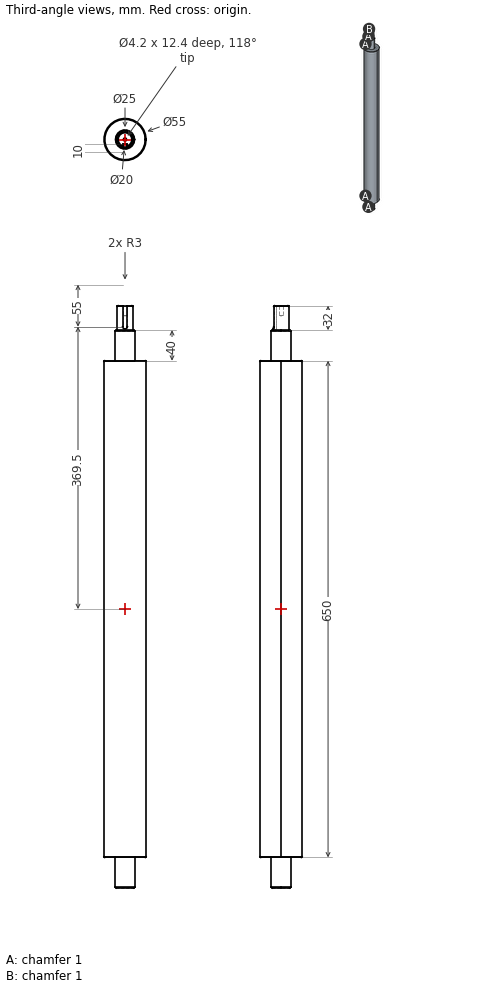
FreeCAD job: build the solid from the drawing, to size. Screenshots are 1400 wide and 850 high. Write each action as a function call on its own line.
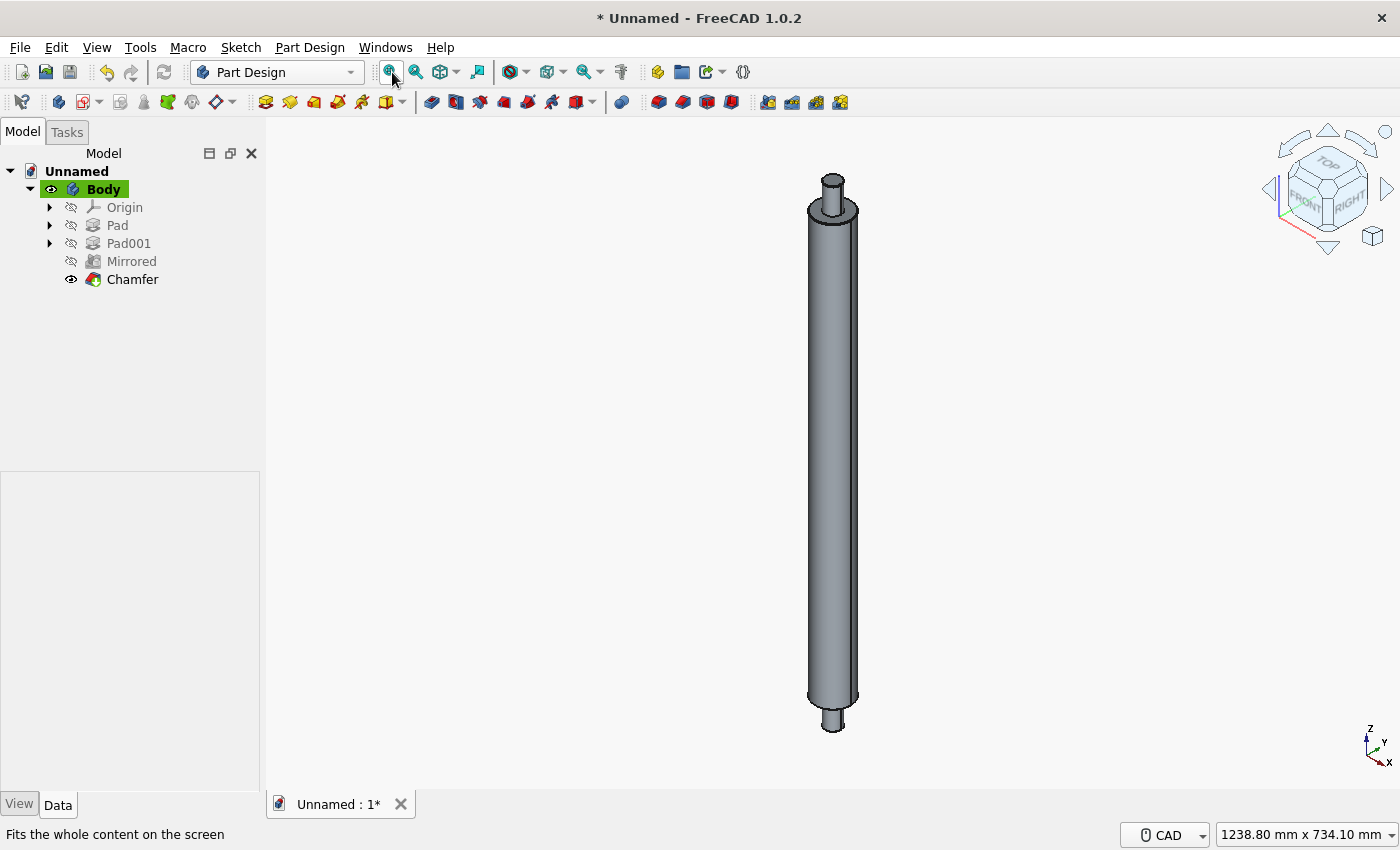
key(2)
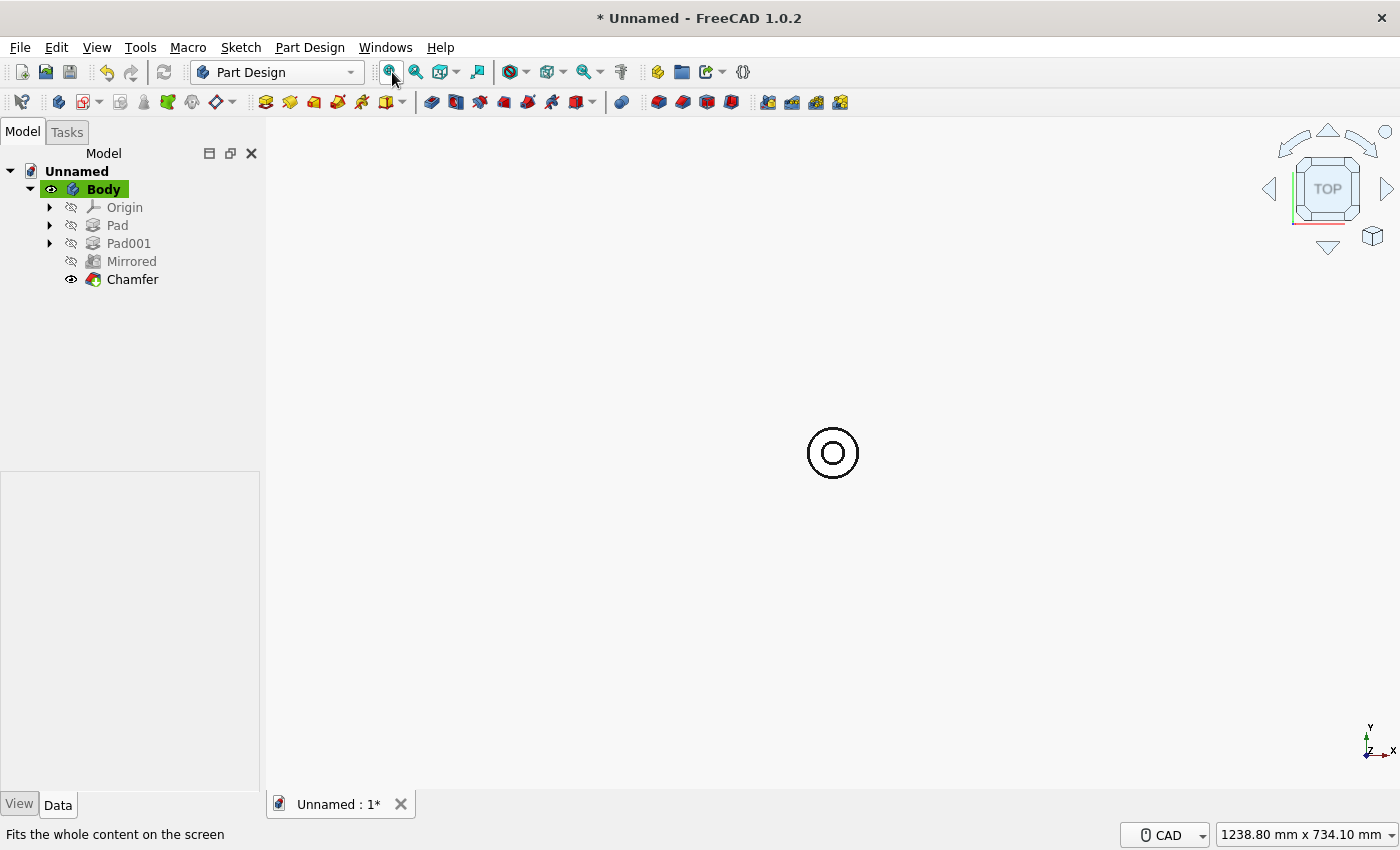
click(392, 72)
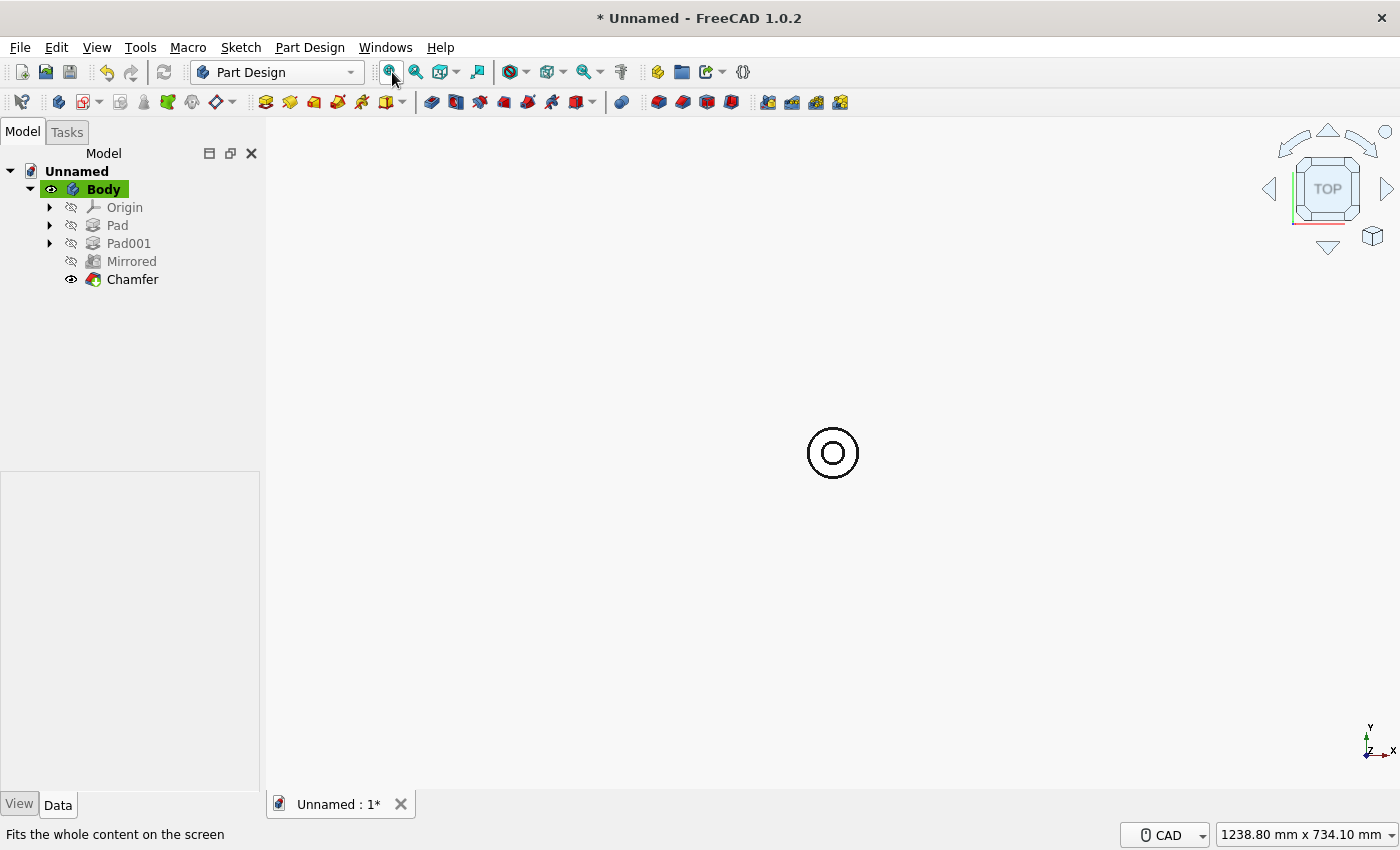
click(833, 452)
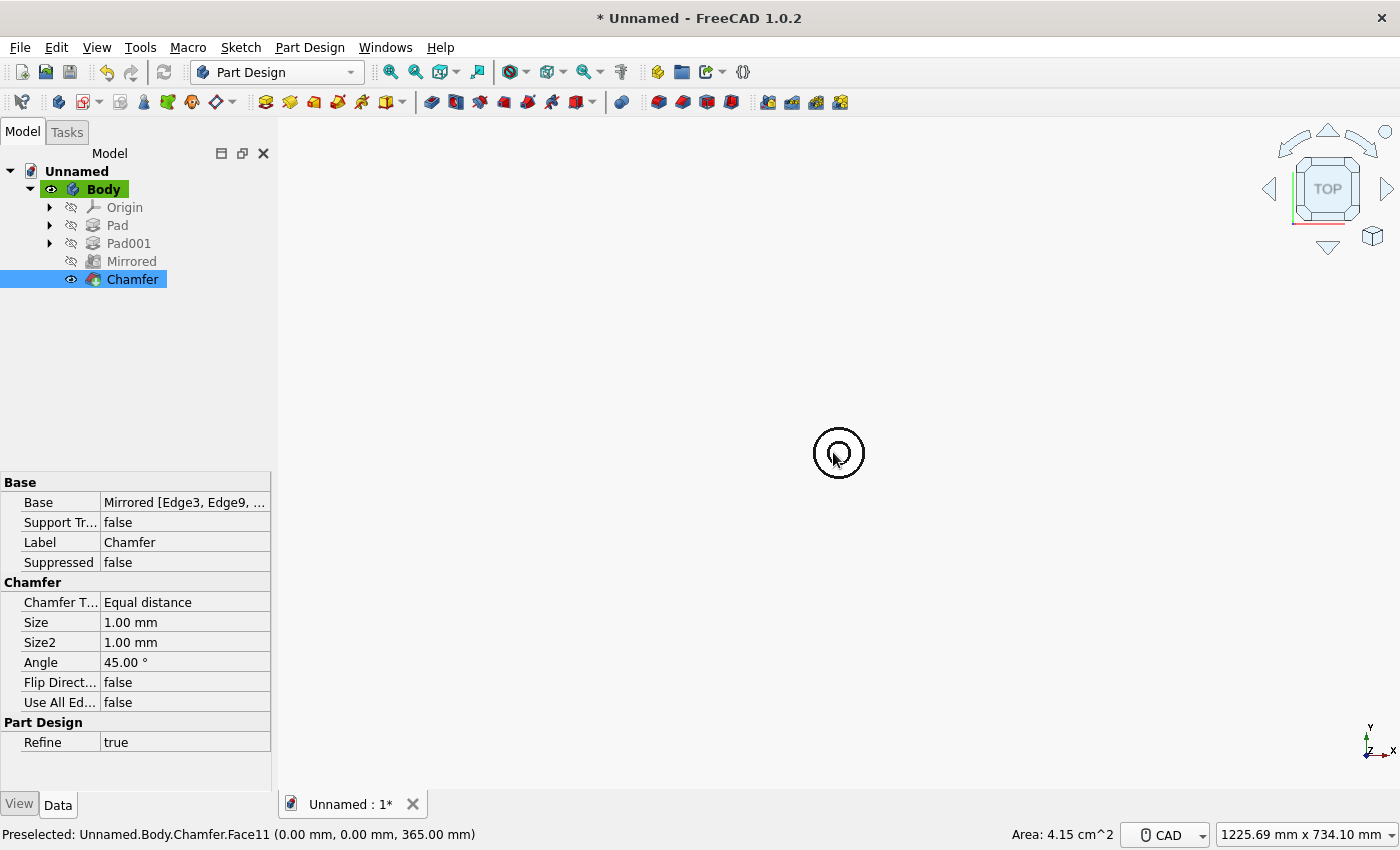
click(84, 102)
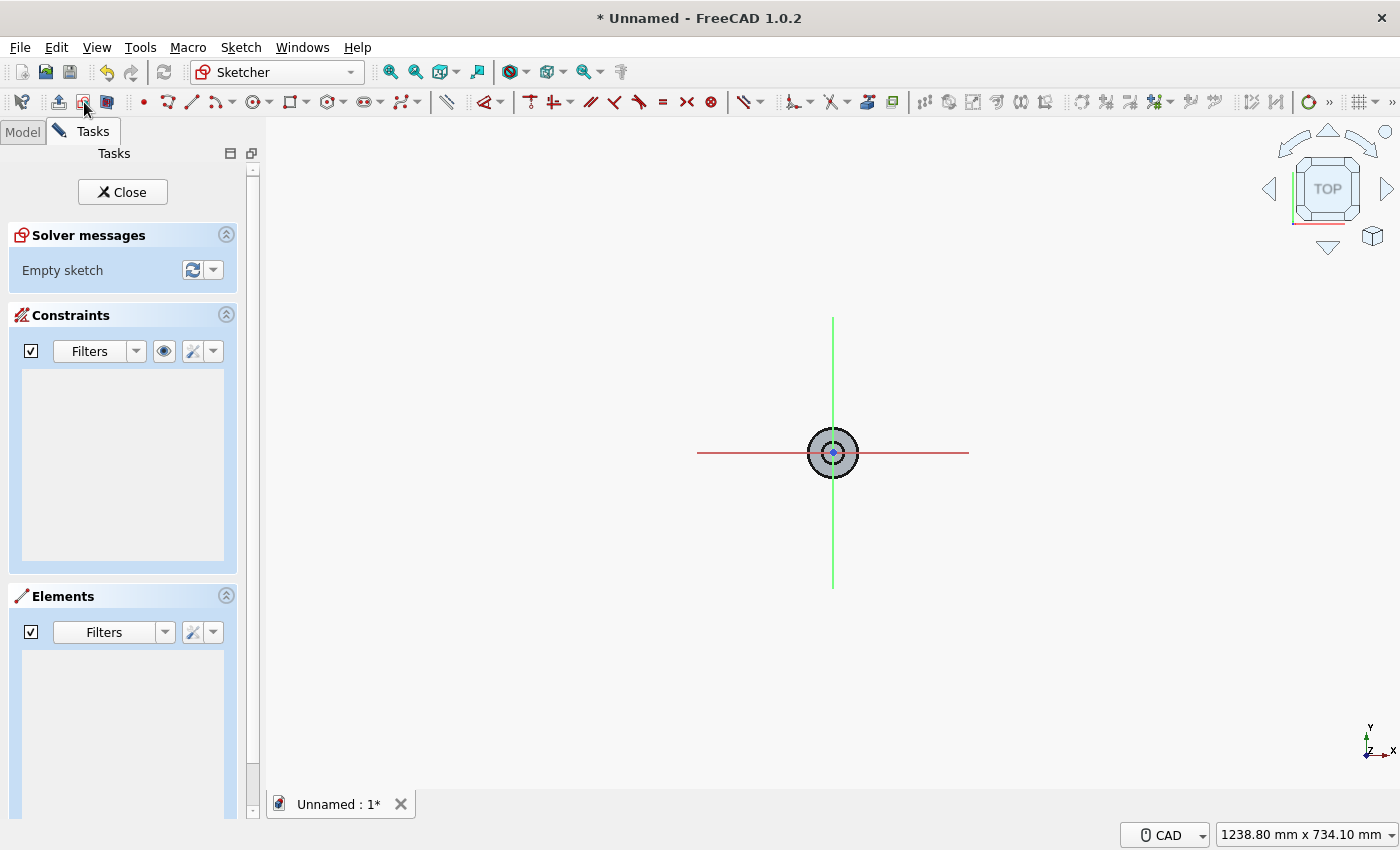
scroll(837, 453, up, 15)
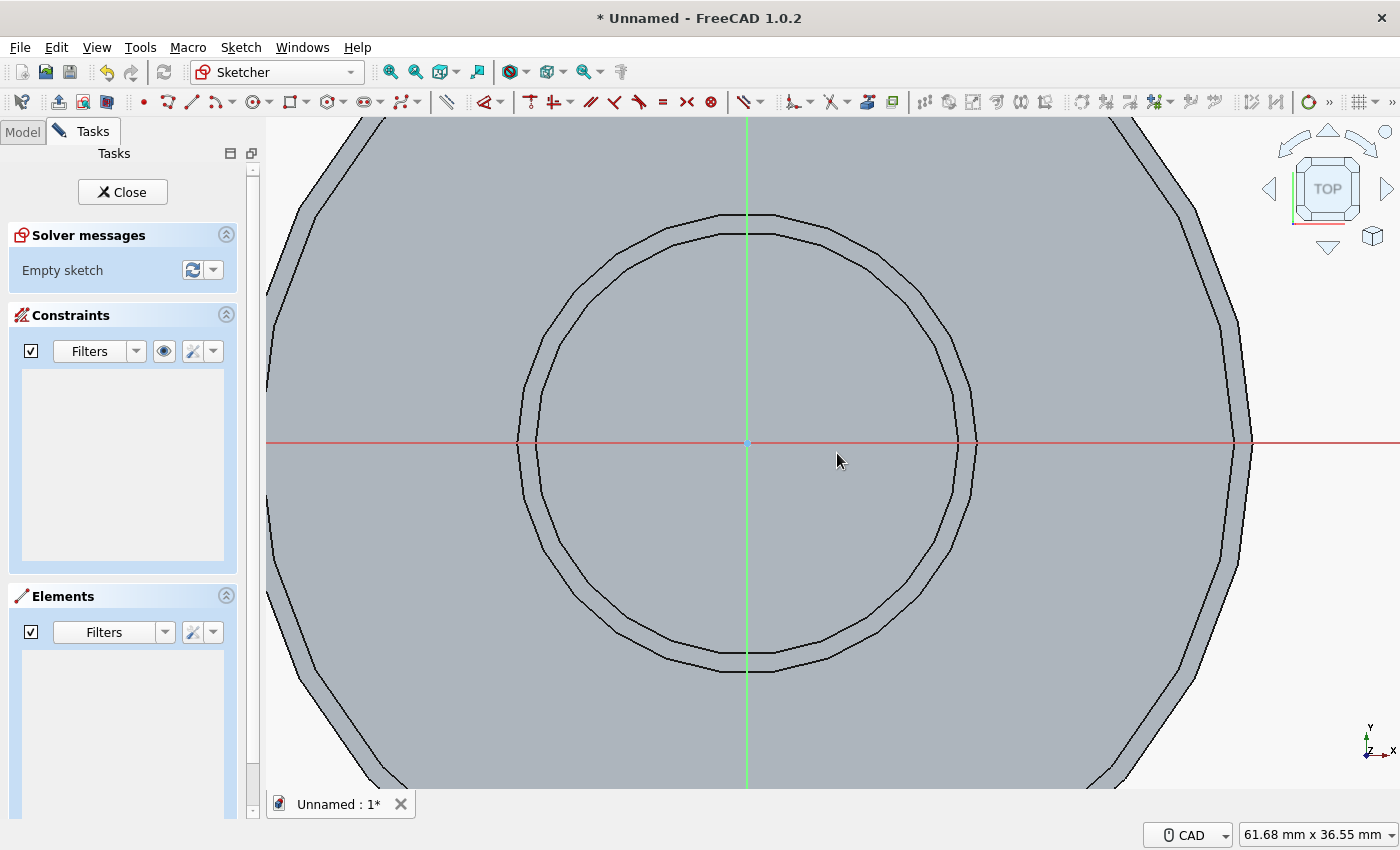
click(254, 102)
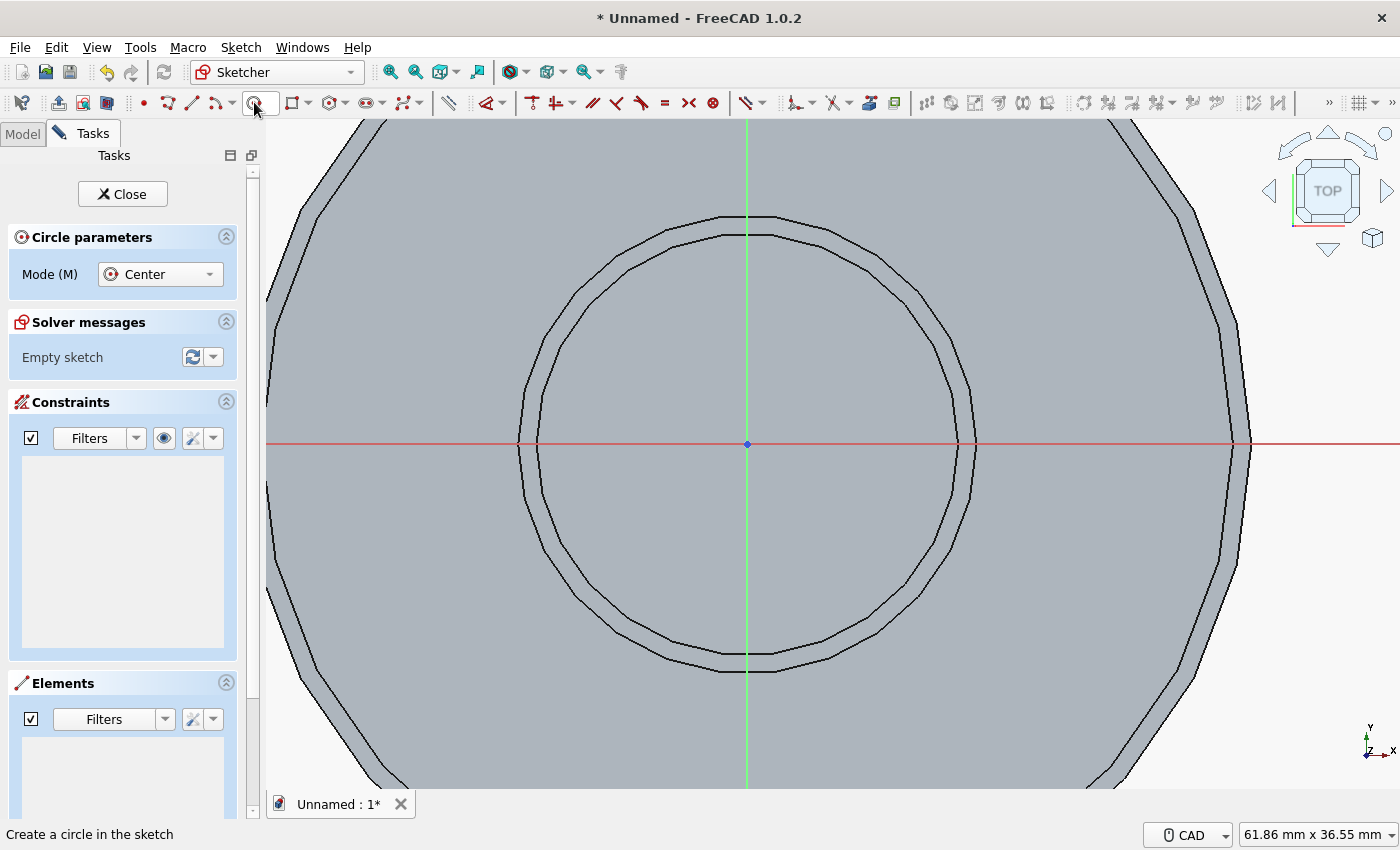
click(747, 444)
move(877, 315)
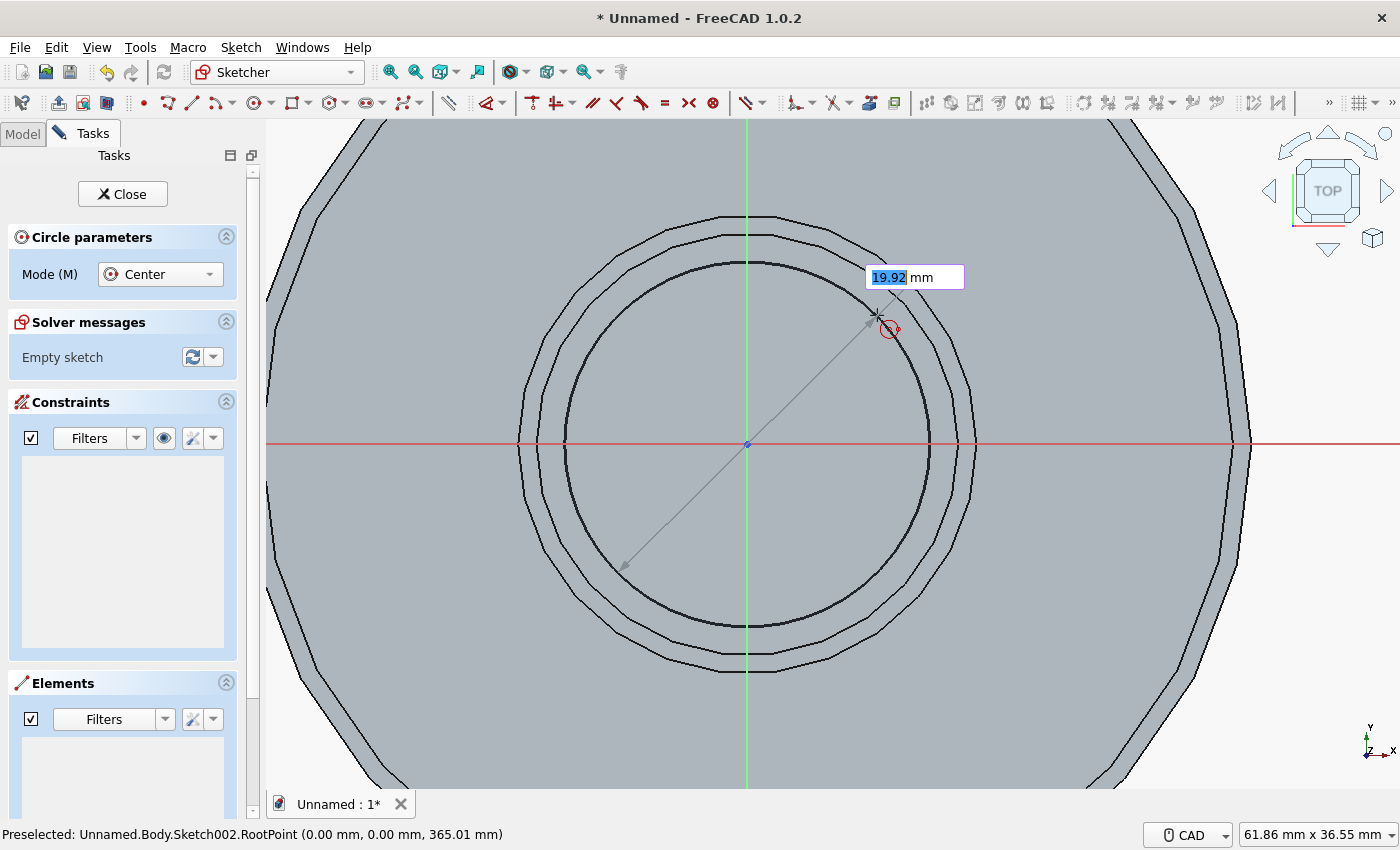
text(20)
key(Return)
key(Escape)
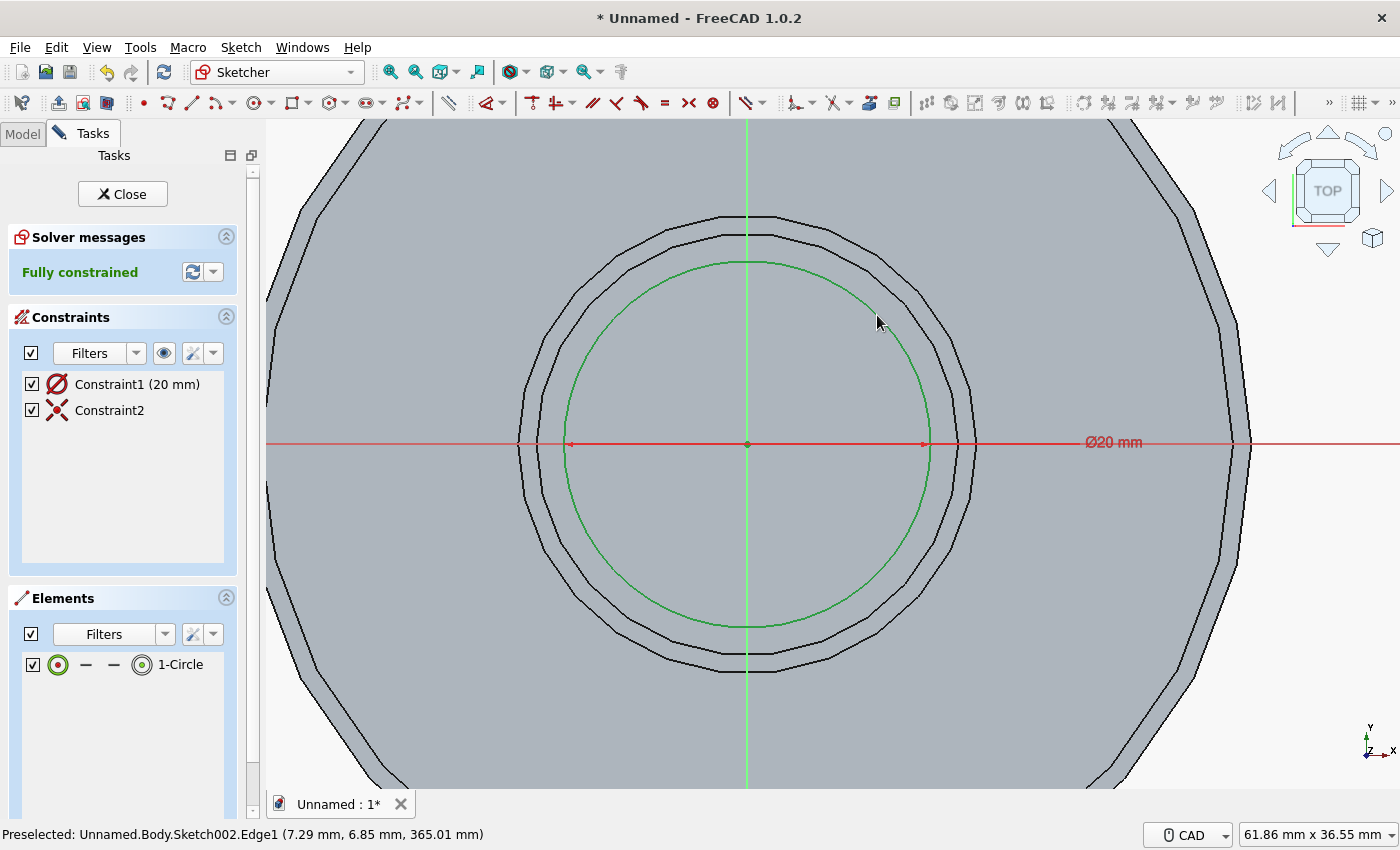
click(123, 194)